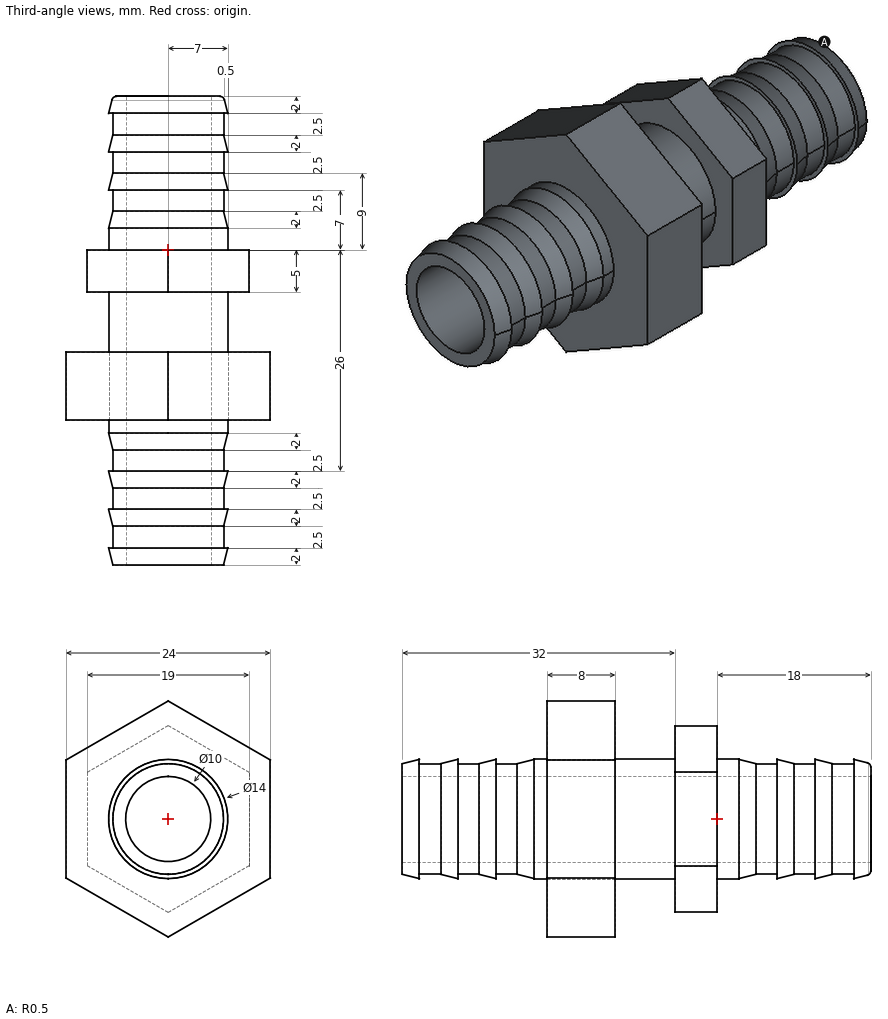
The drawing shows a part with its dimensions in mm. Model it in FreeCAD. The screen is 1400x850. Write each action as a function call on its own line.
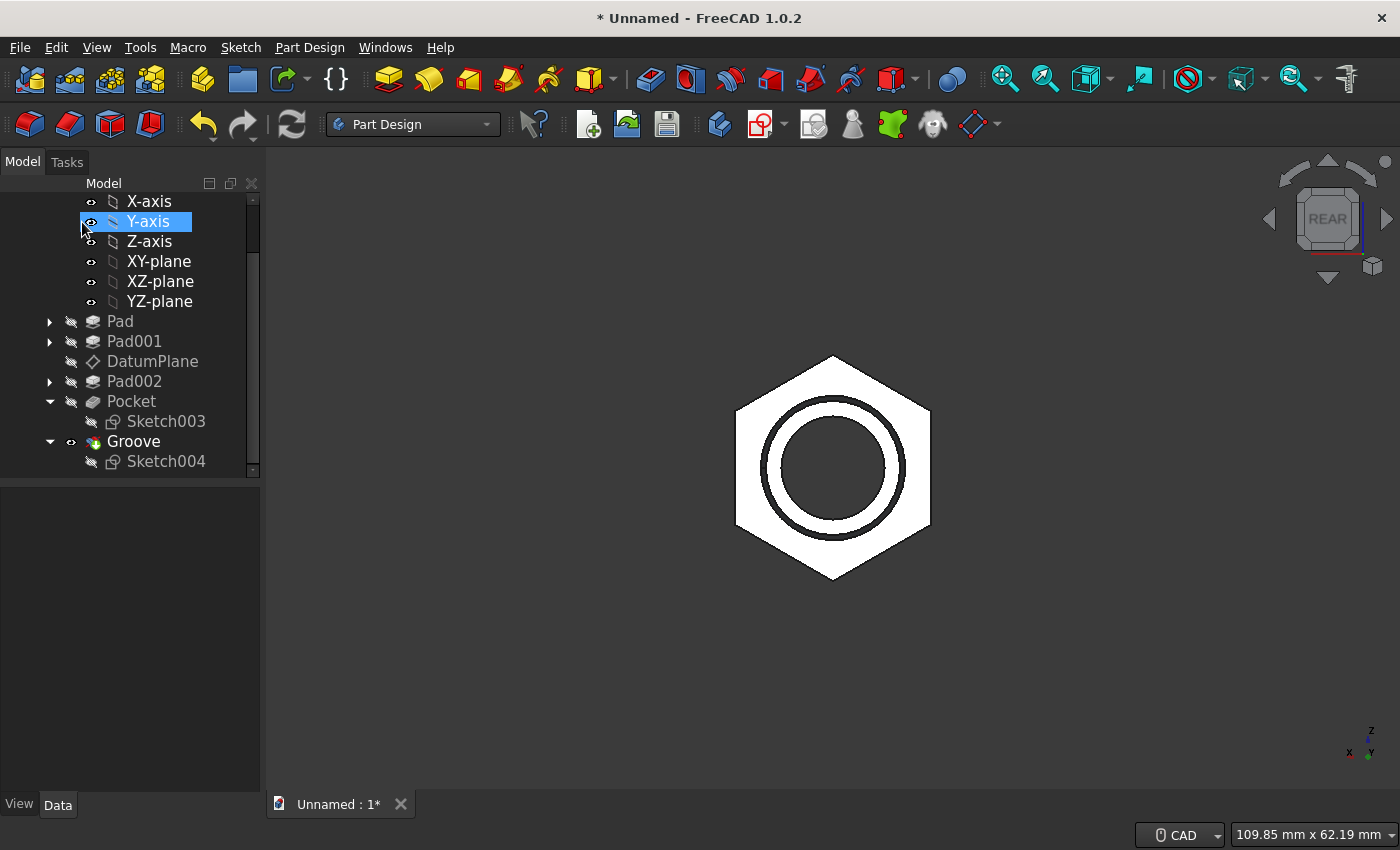
click(1006, 80)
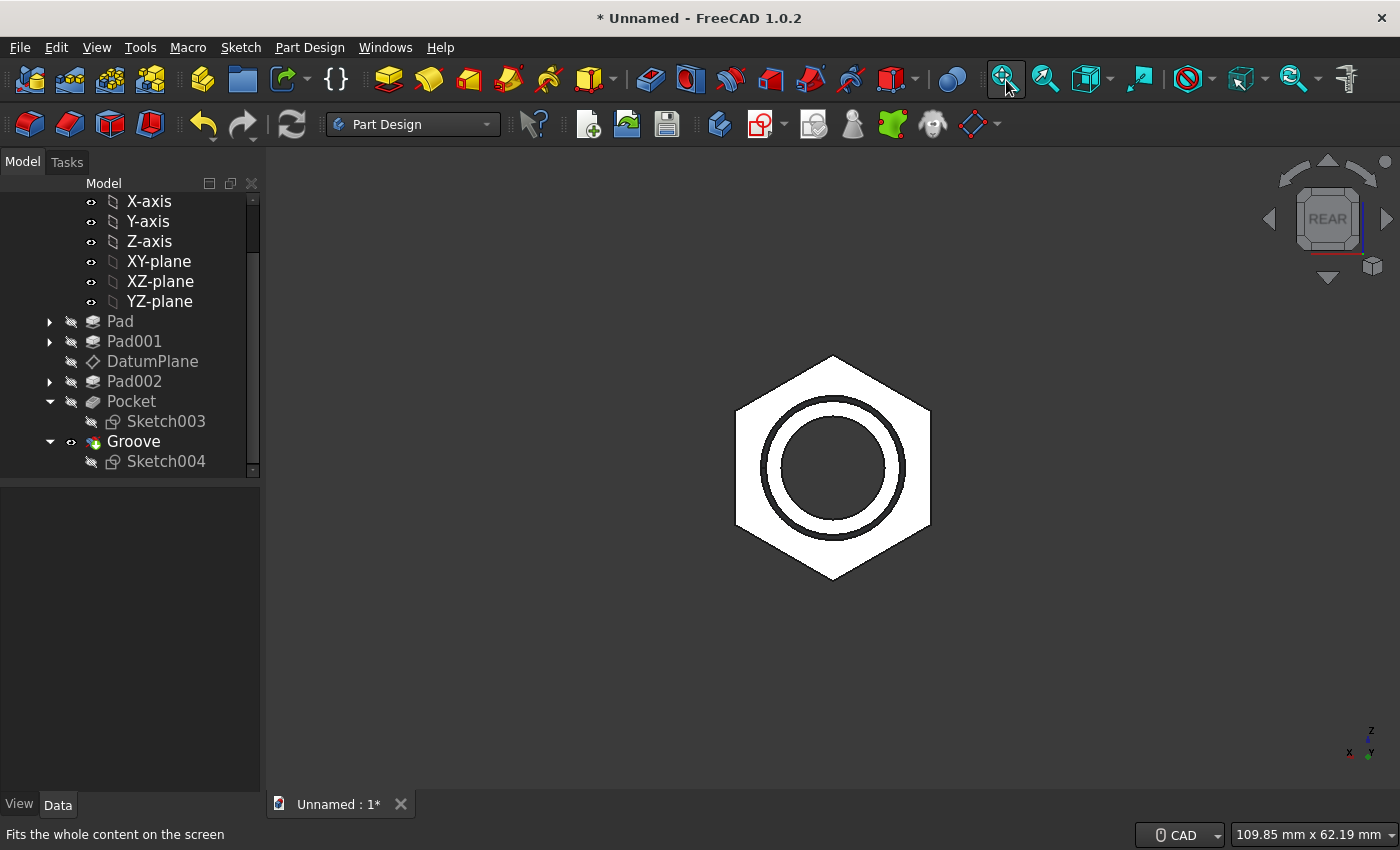
click(900, 467)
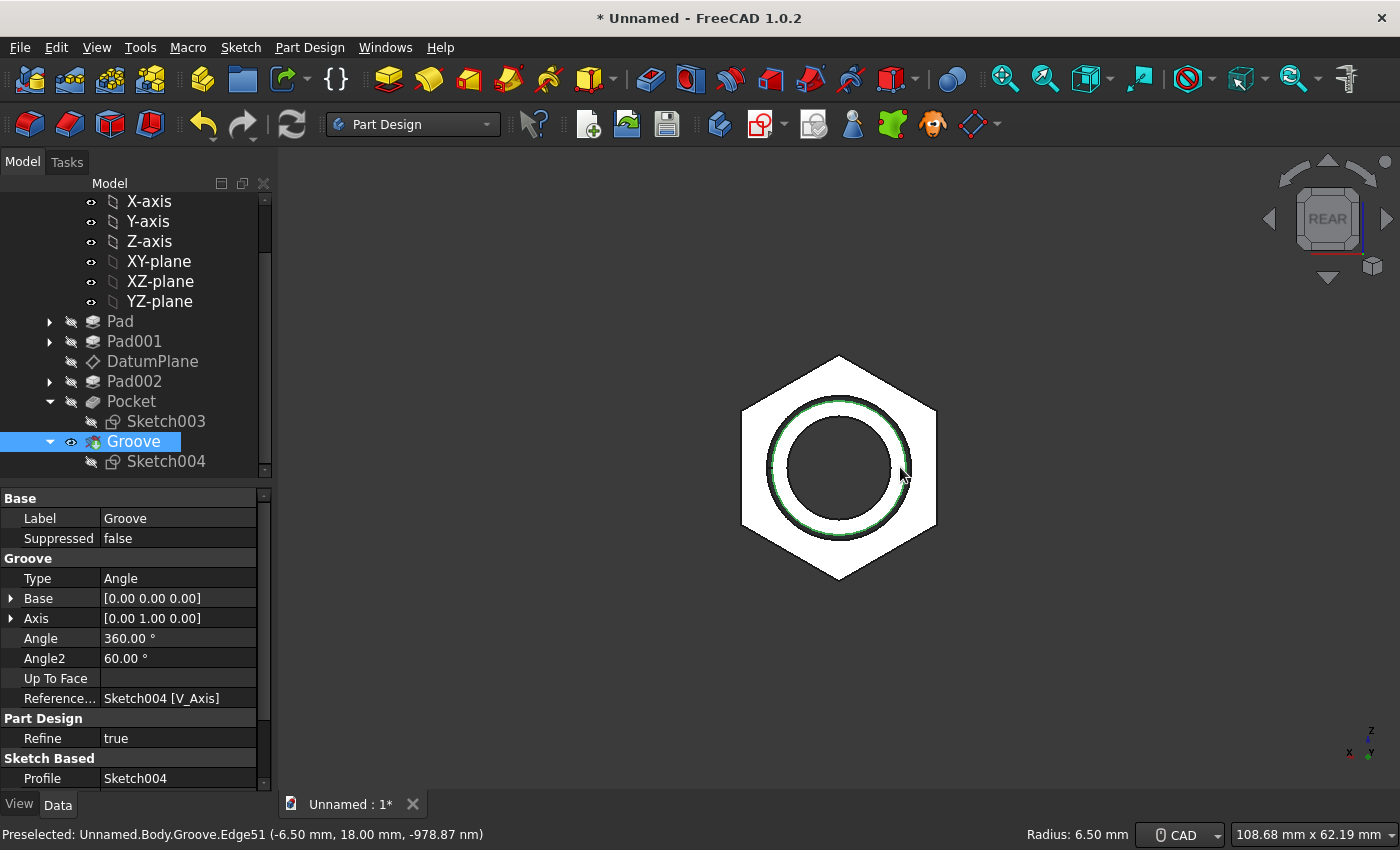
click(30, 124)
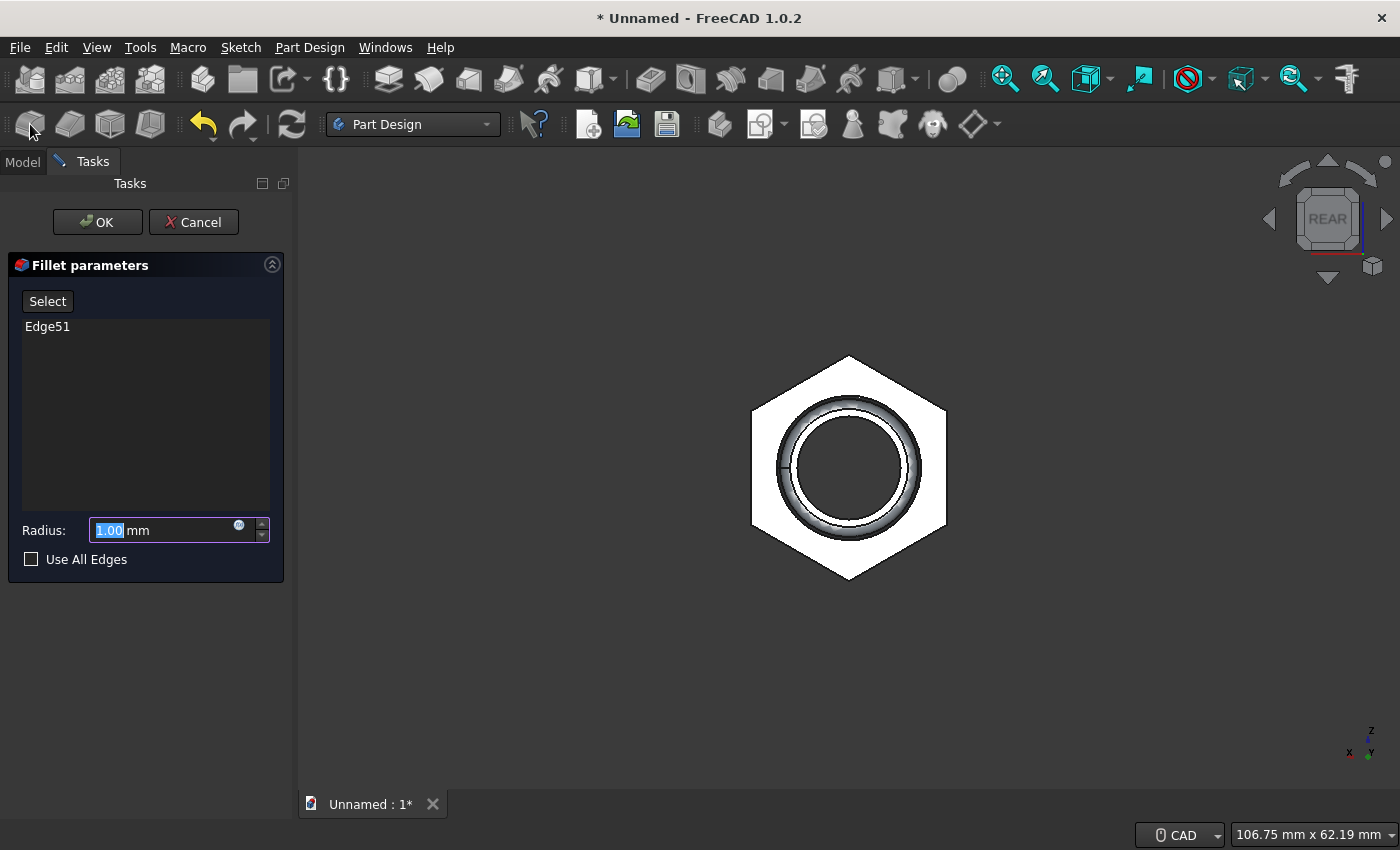
text(0.5)
key(Tab)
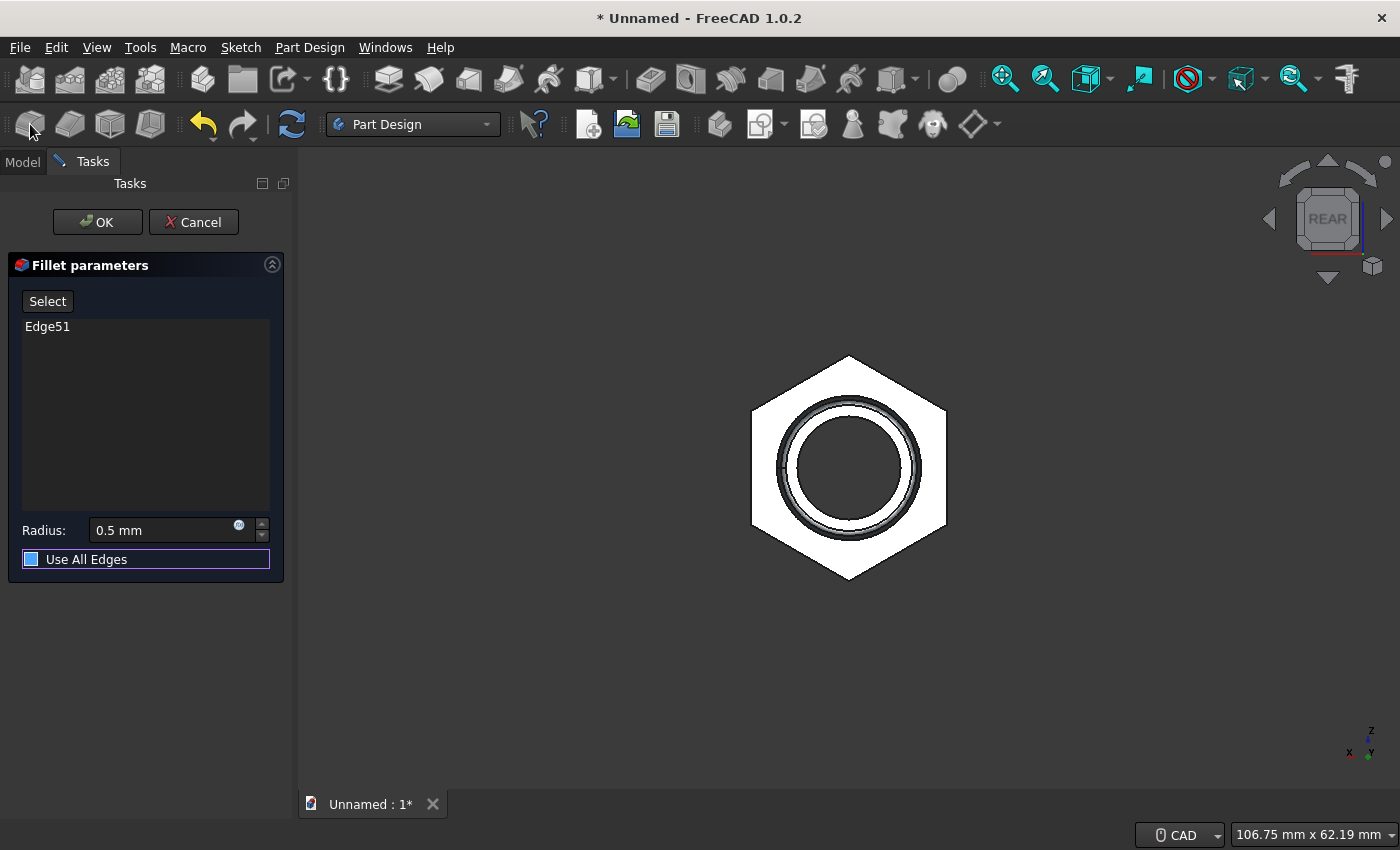
click(98, 222)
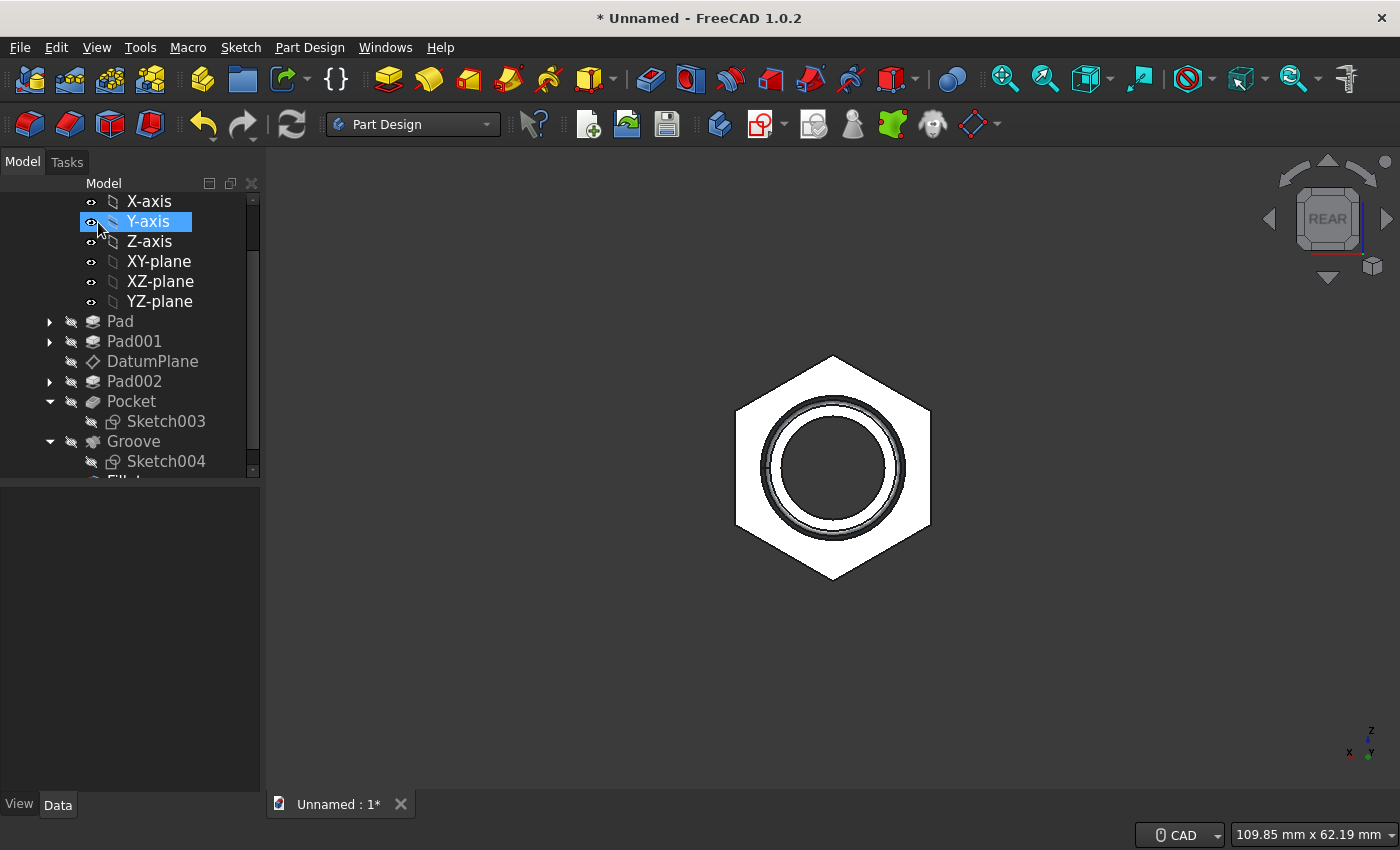
click(1006, 80)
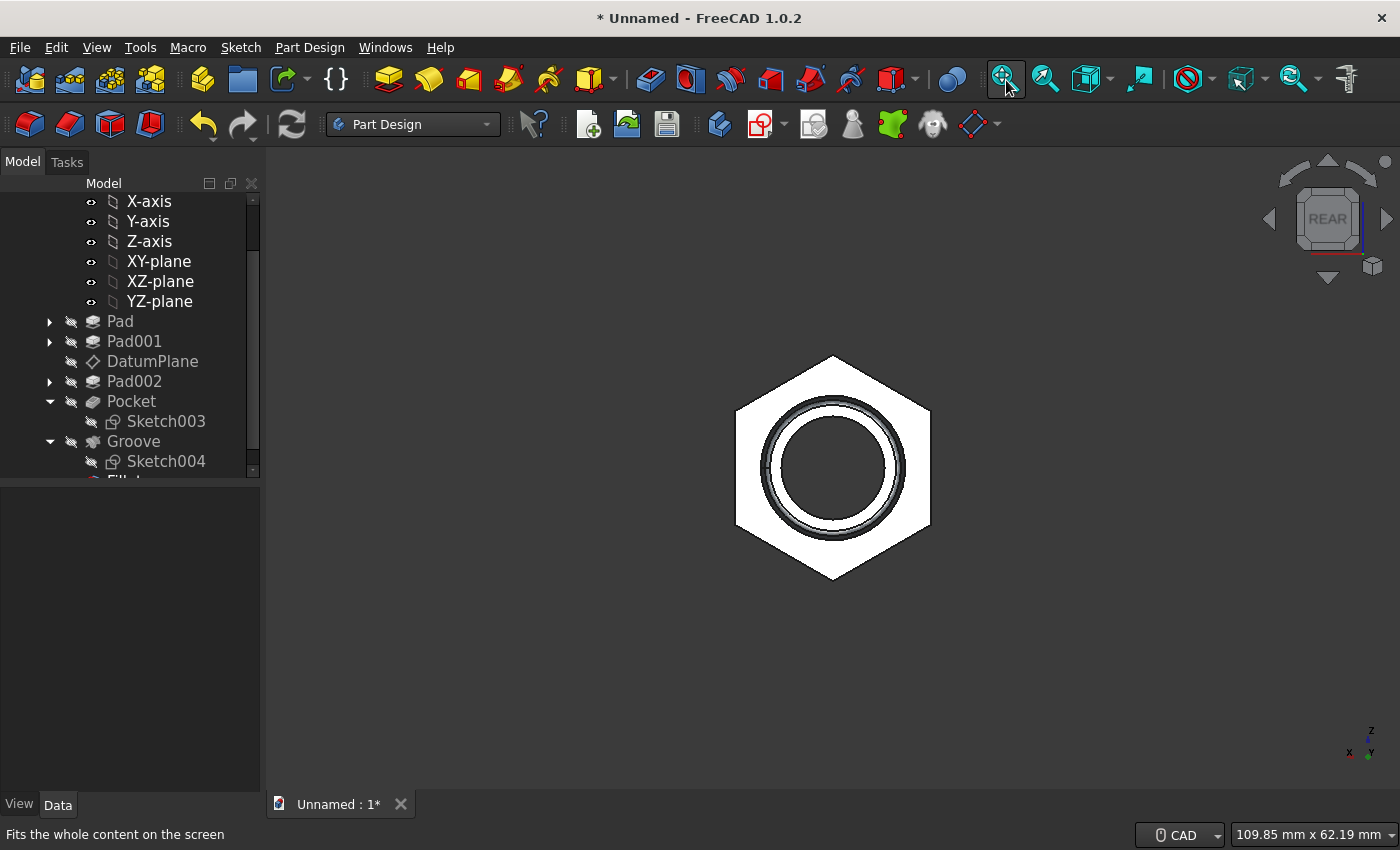
click(720, 124)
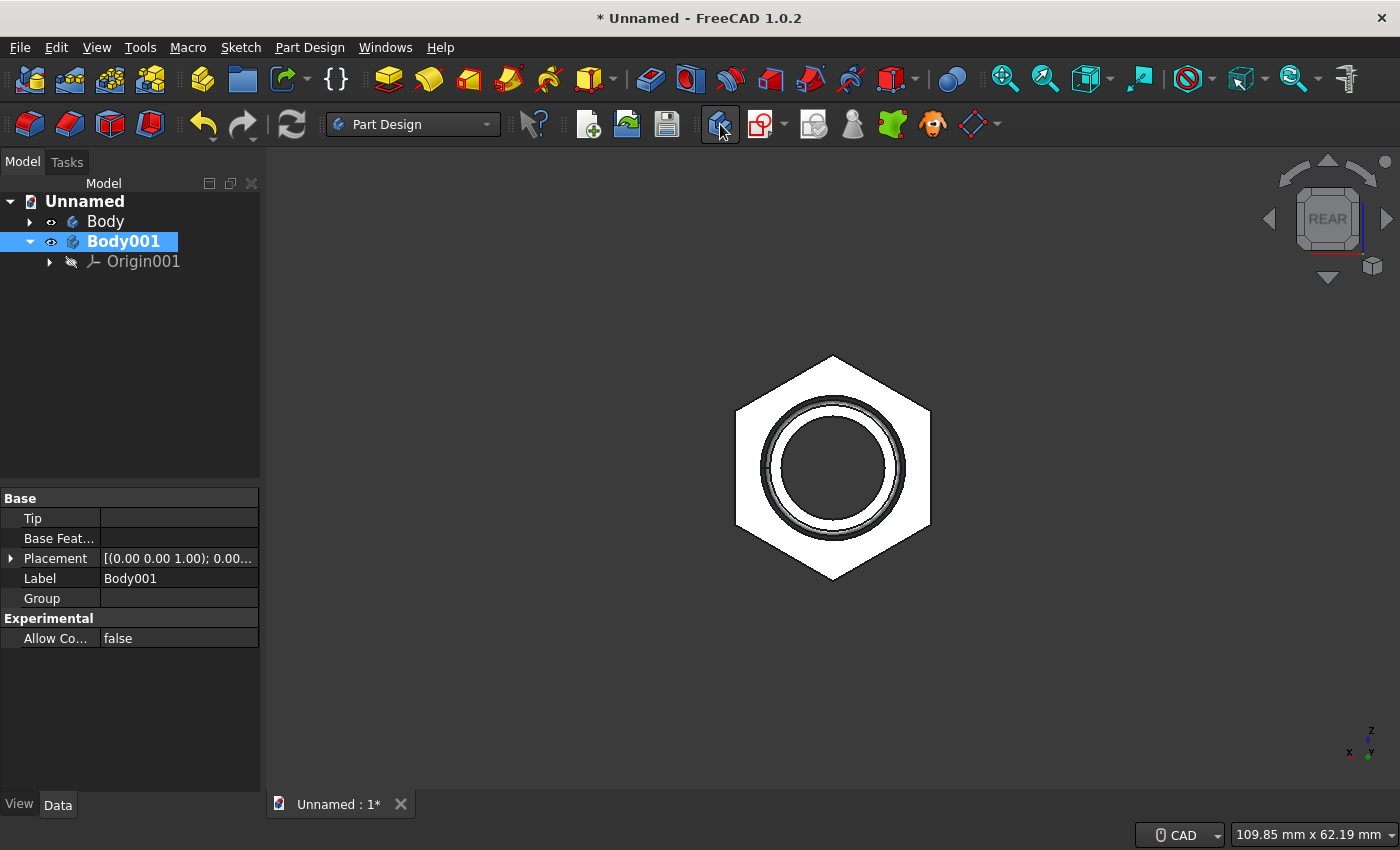
click(50, 262)